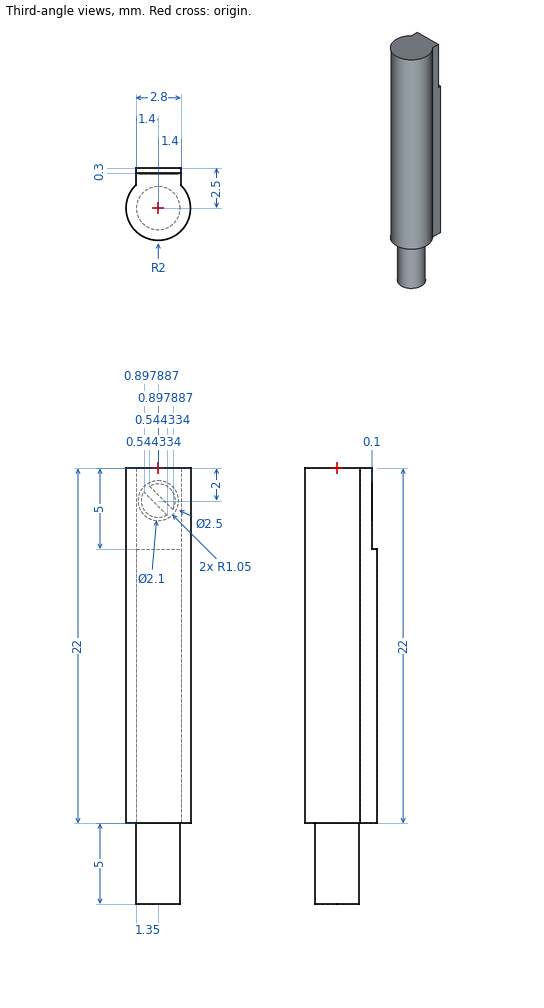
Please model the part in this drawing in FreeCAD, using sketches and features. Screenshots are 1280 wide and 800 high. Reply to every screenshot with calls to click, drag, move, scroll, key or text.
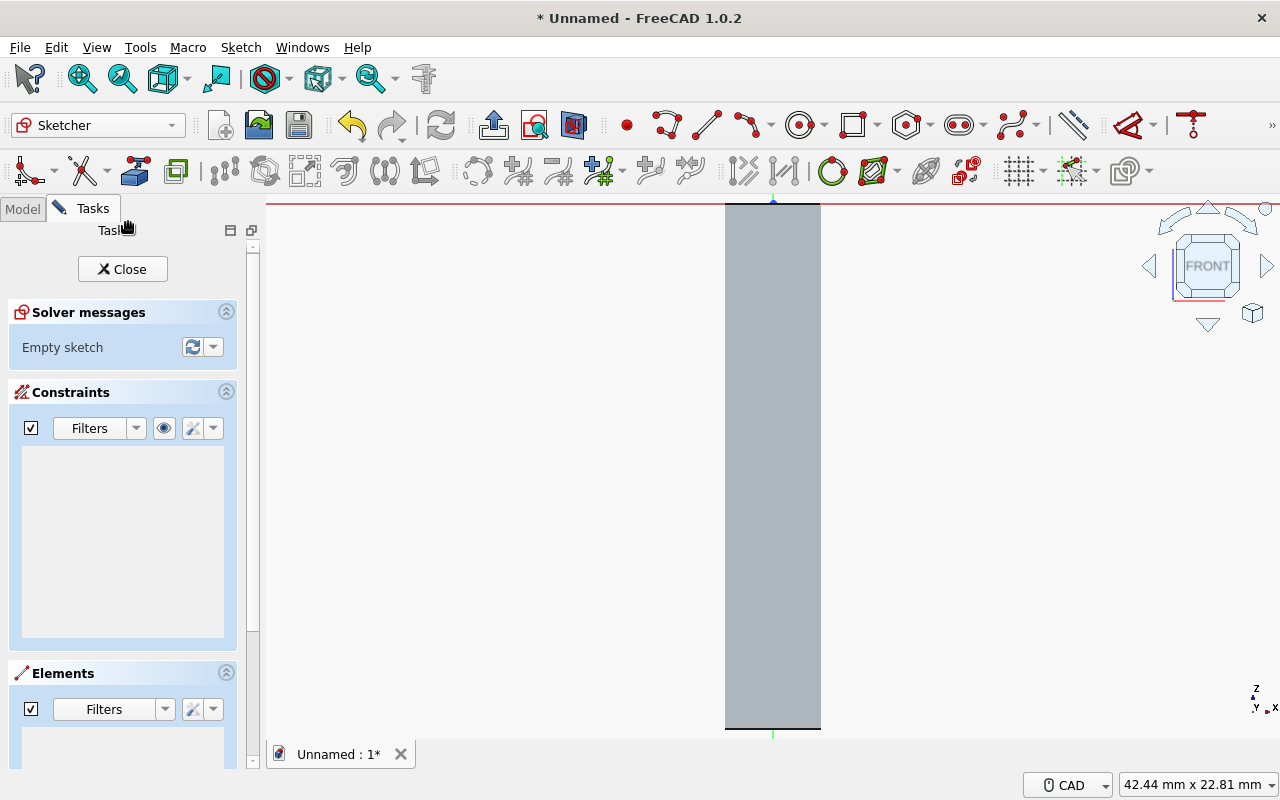
click(574, 126)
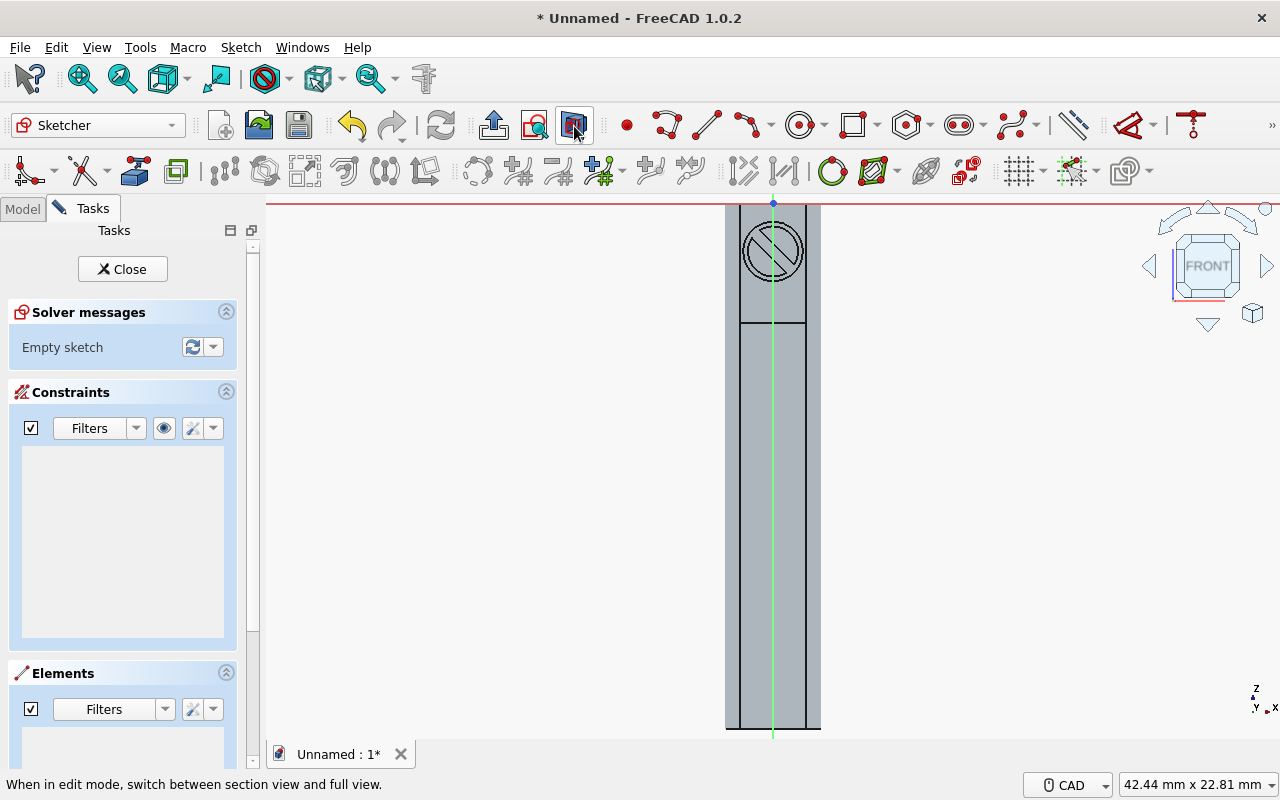
scroll(704, 466, down, 5)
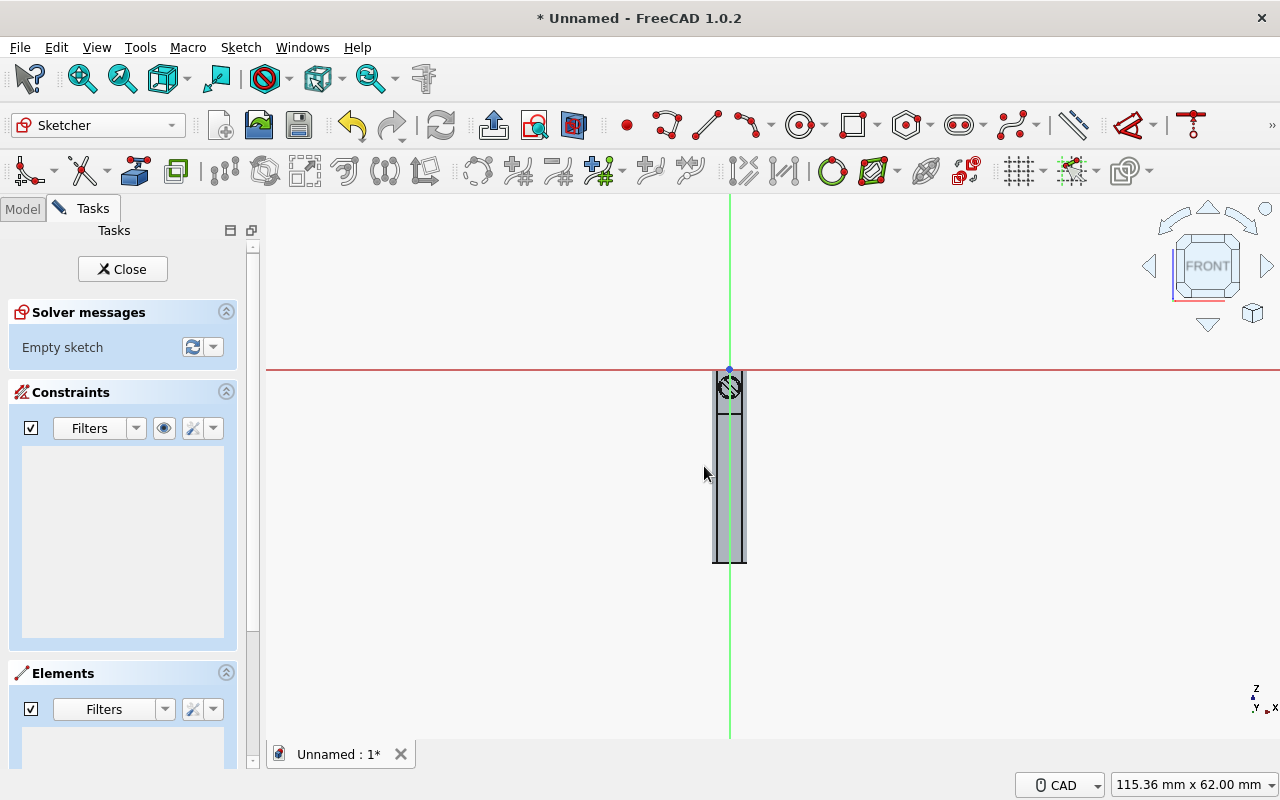
scroll(727, 604, up, 10)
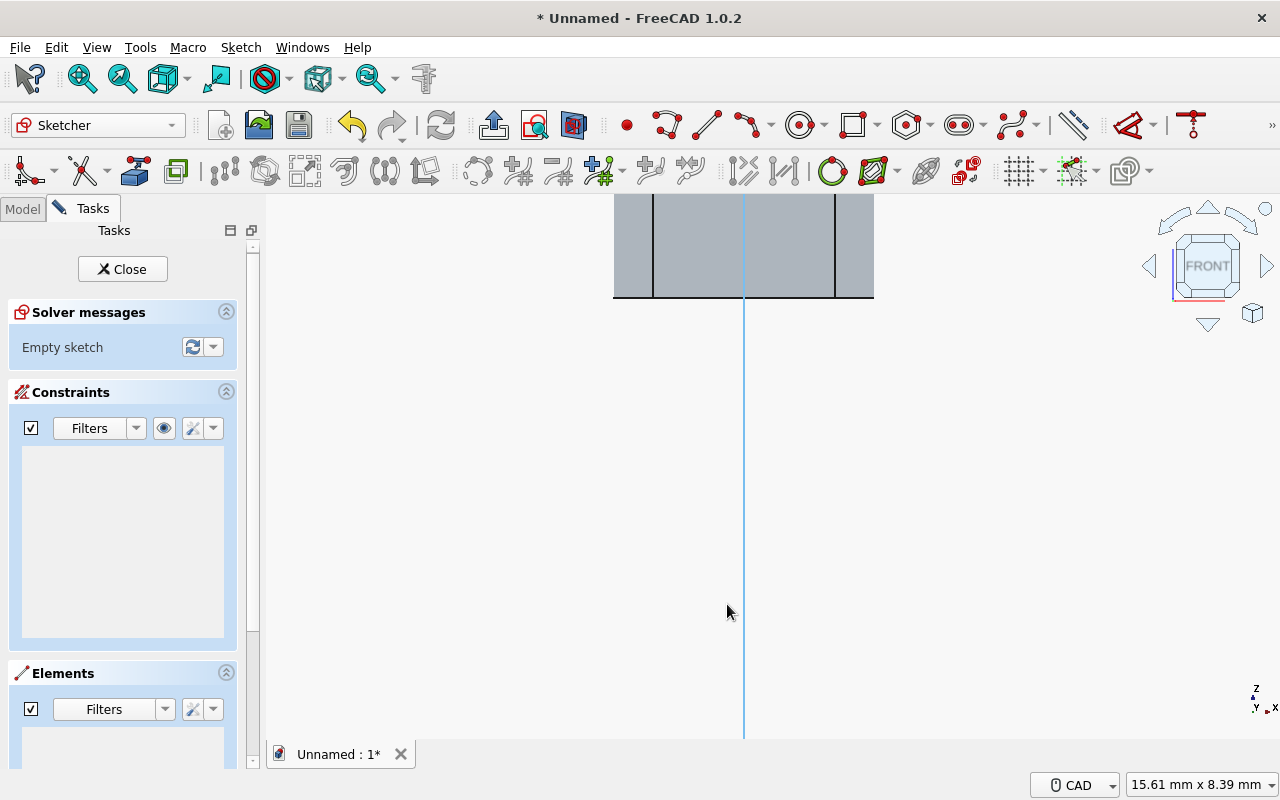
click(854, 126)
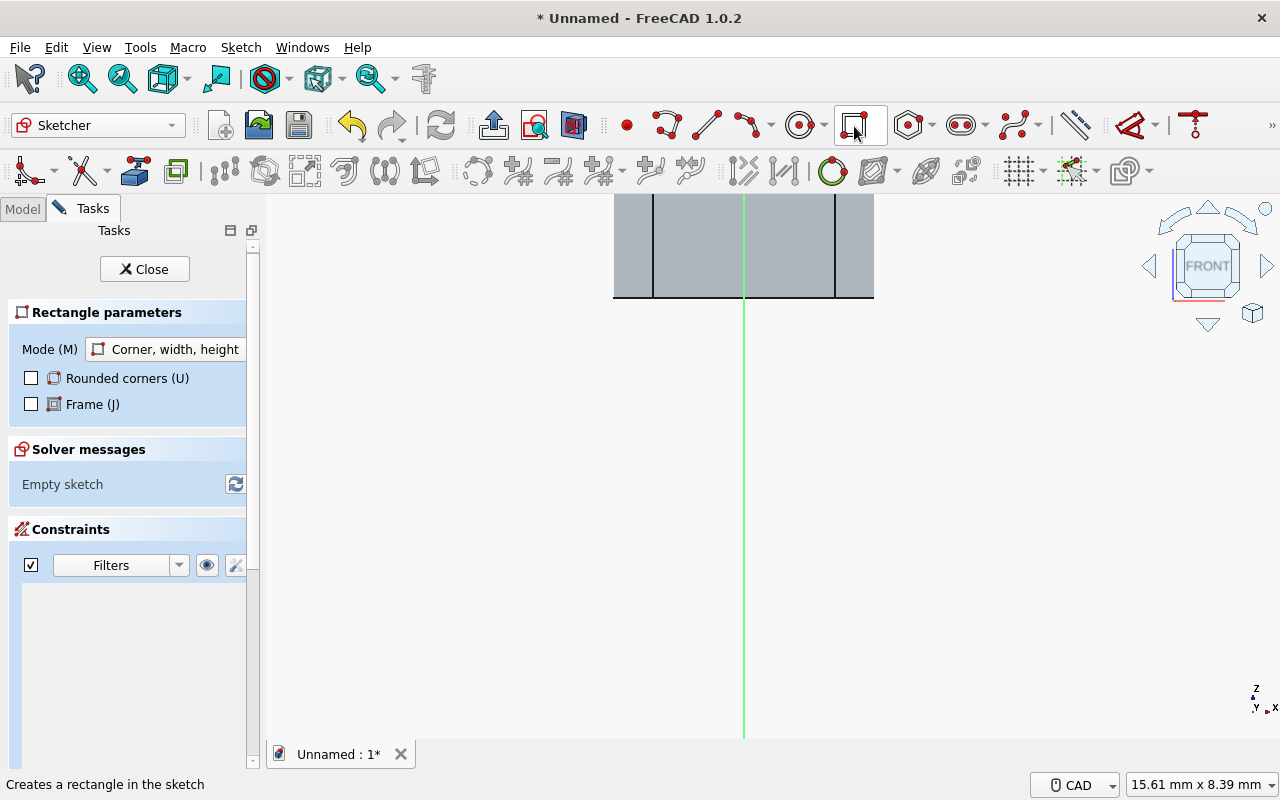
click(656, 298)
click(744, 622)
key(Escape)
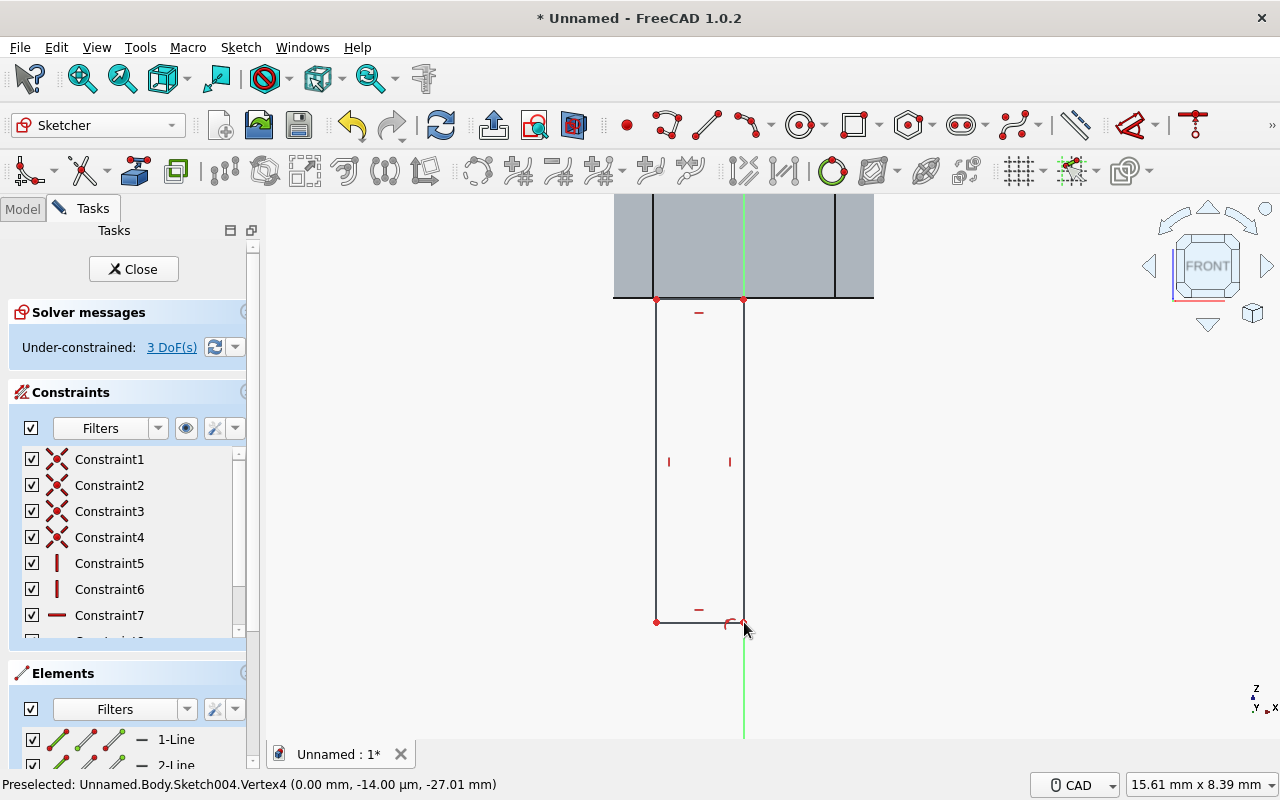
click(1130, 126)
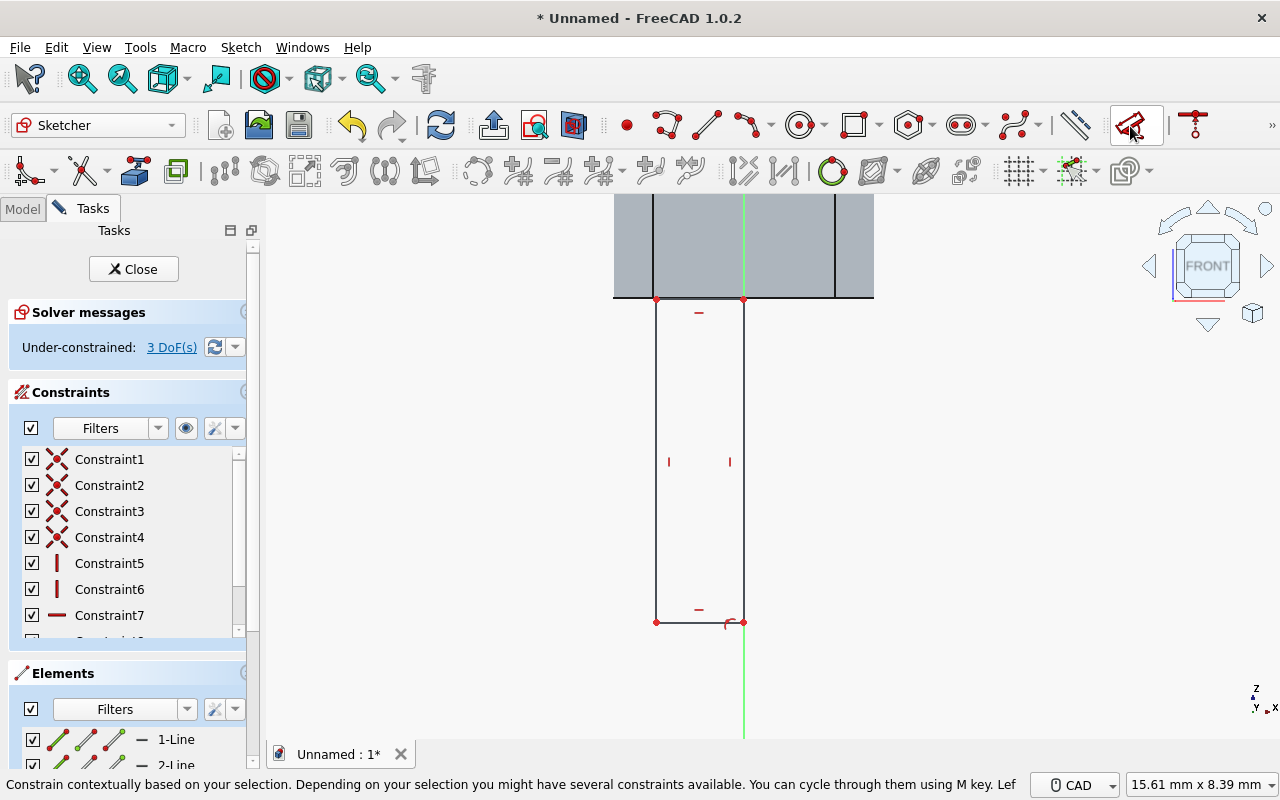
click(656, 396)
click(622, 461)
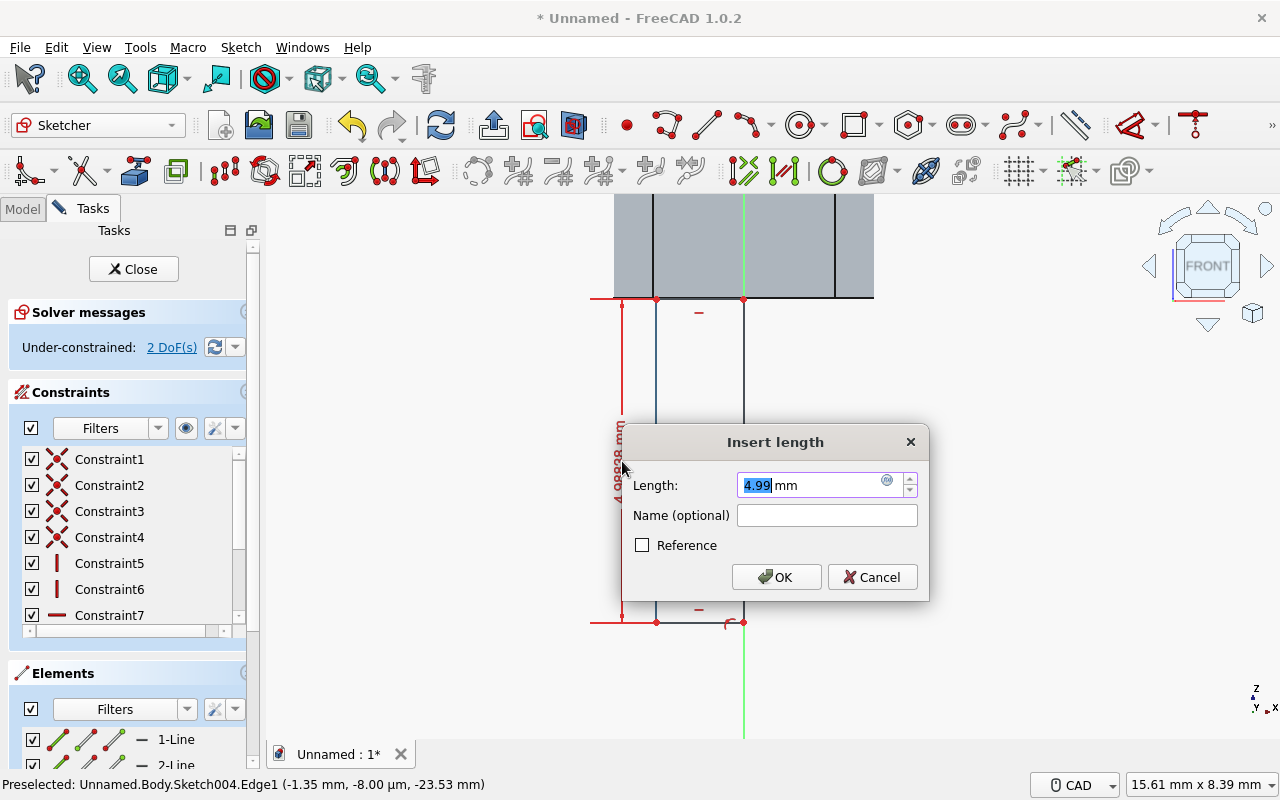
text(5)
key(Return)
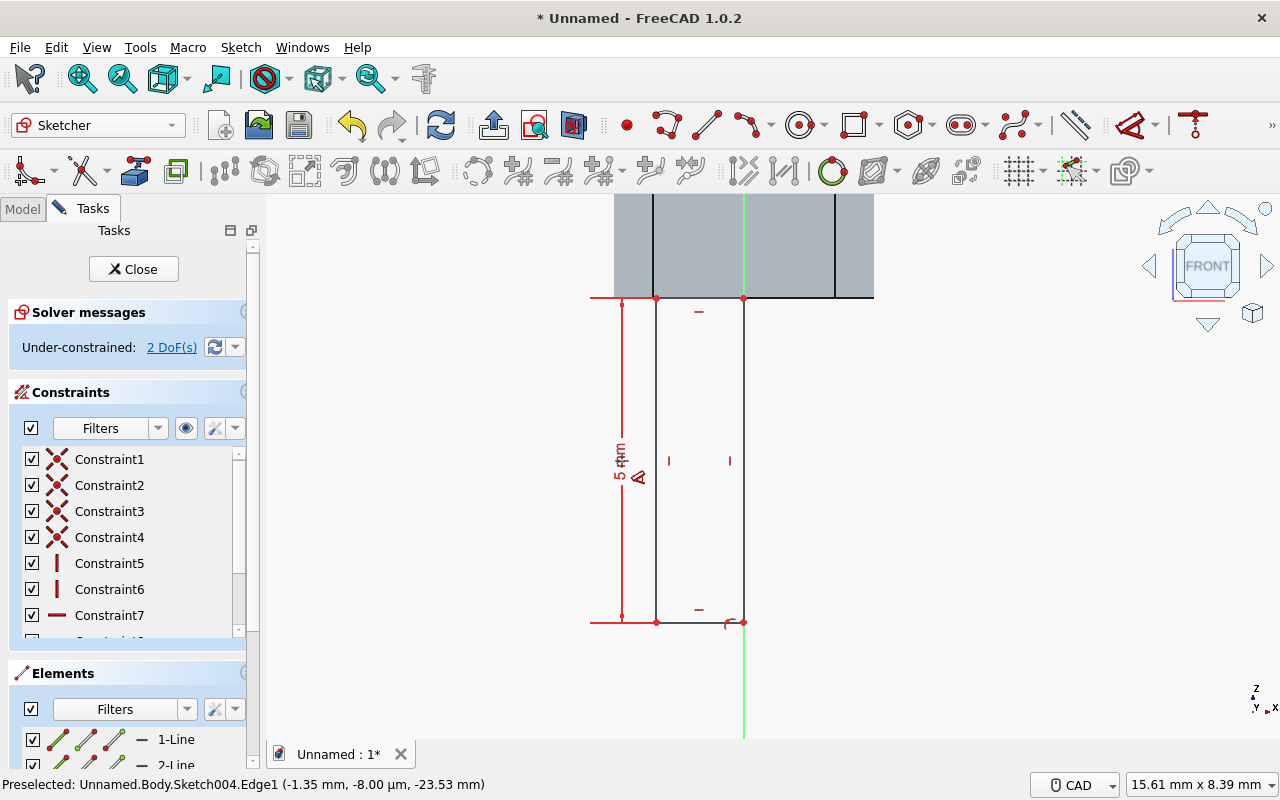
click(656, 298)
click(622, 260)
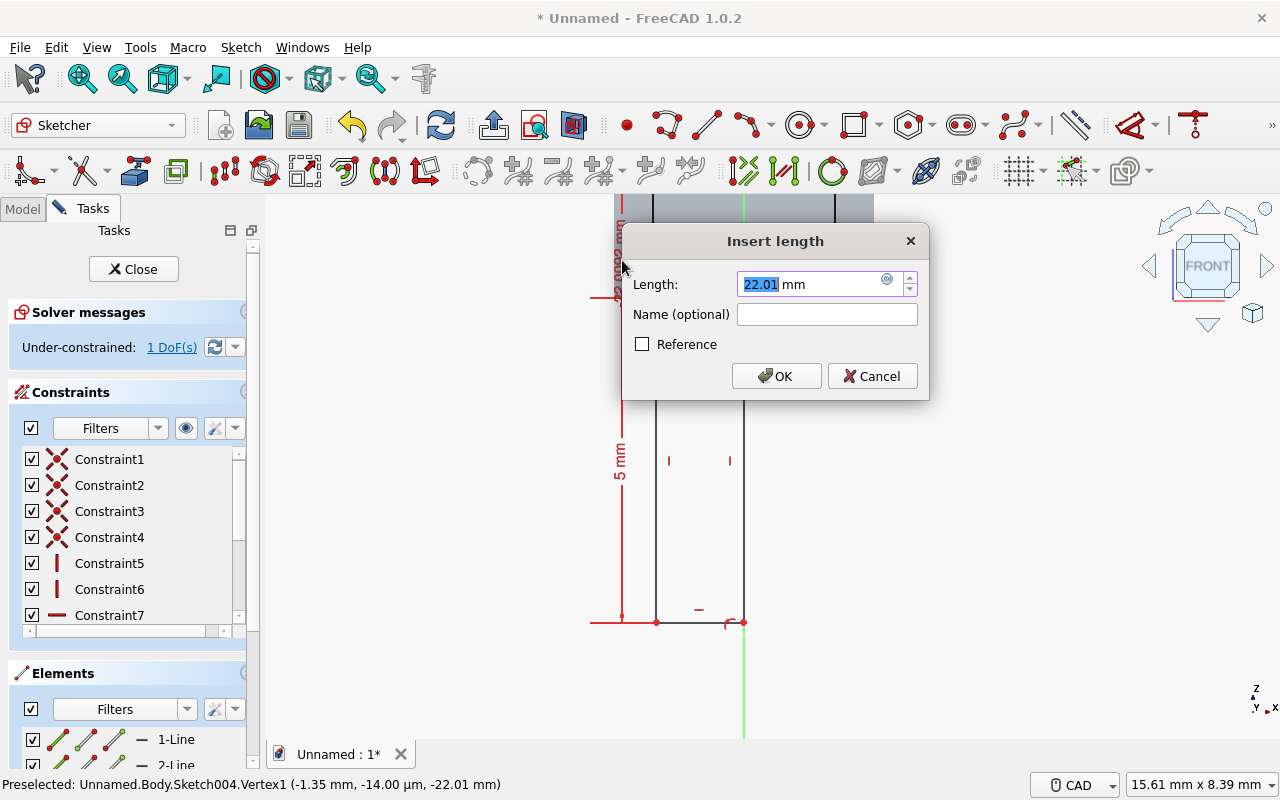
text(22)
key(Return)